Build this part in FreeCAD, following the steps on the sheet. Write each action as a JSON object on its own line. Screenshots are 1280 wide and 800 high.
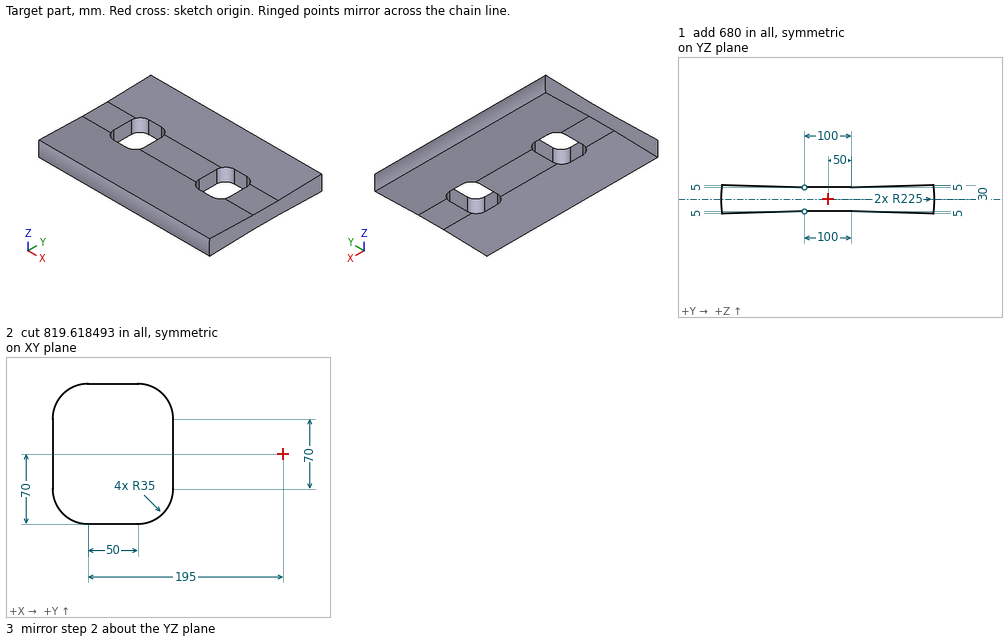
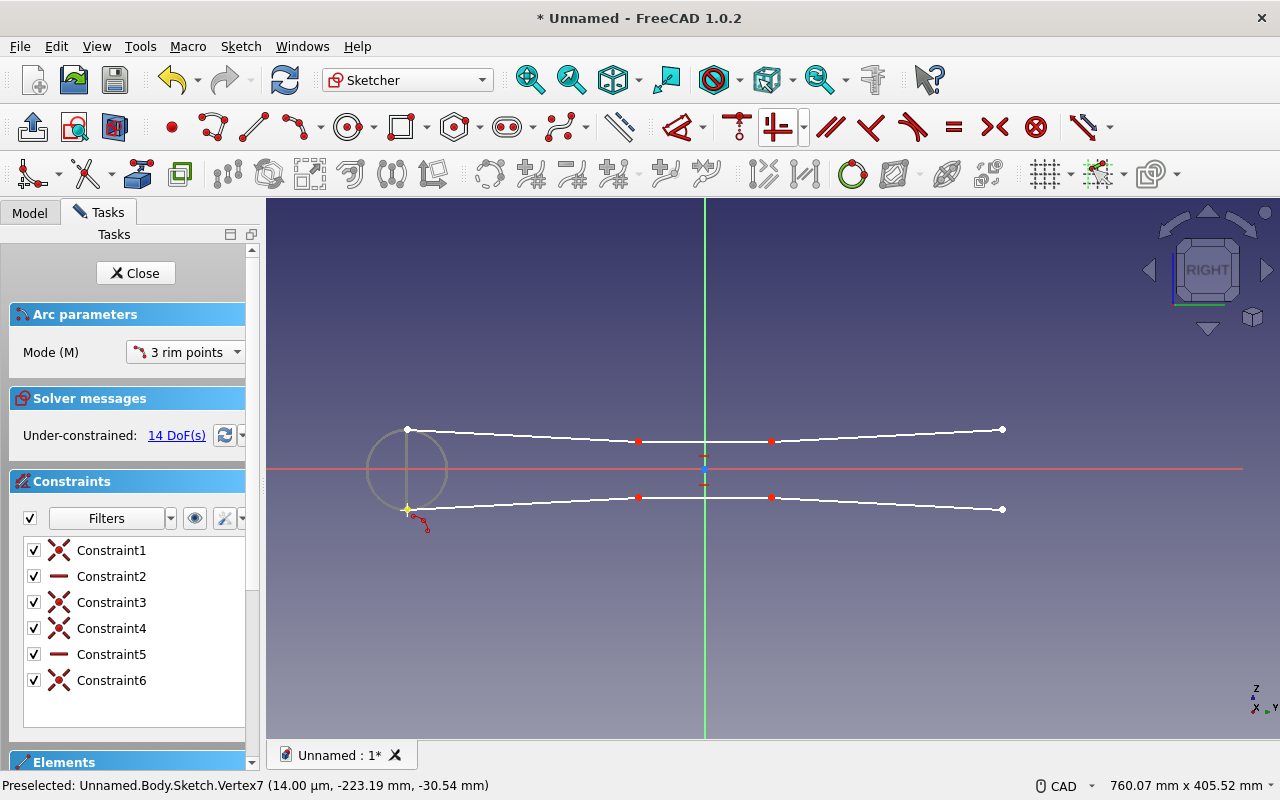
{"action": "scroll", "coordinate": [405, 461], "scroll_direction": "up", "scroll_amount": 10}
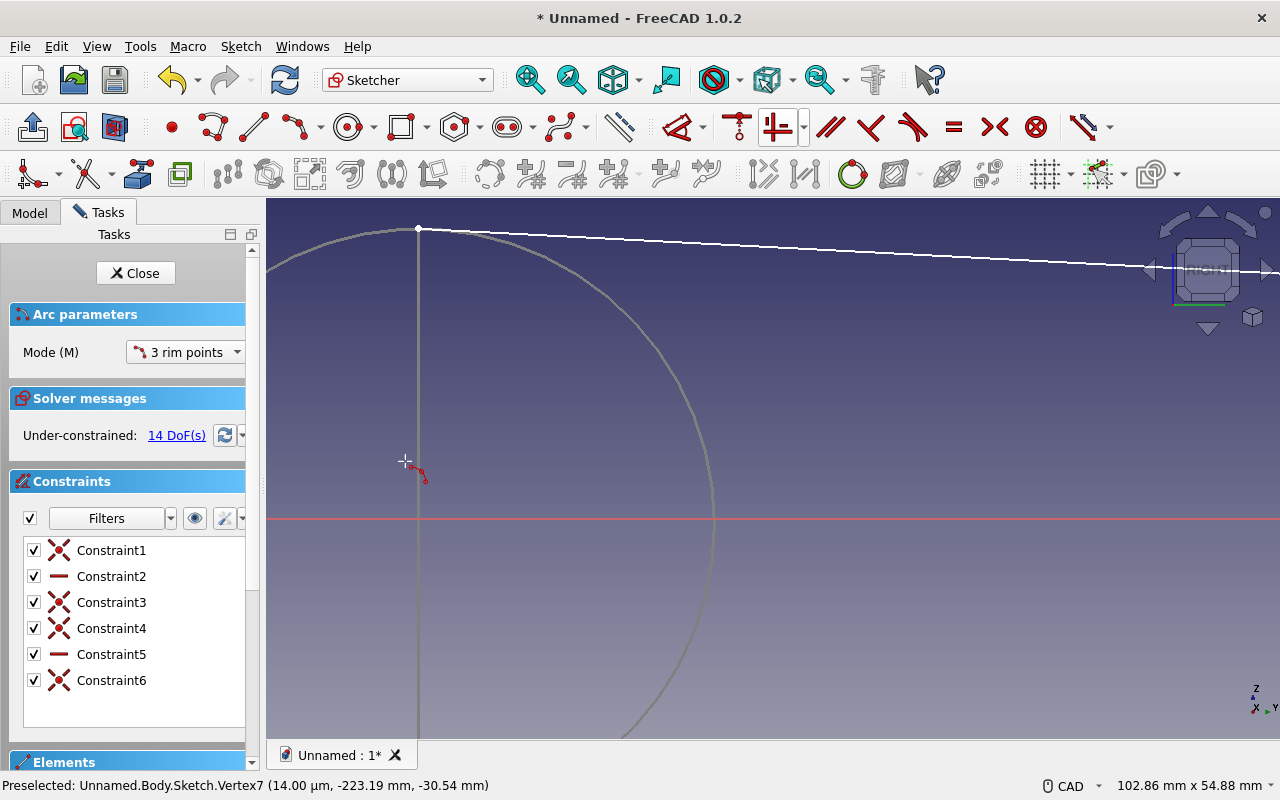
{"action": "left_click", "coordinate": [402, 460]}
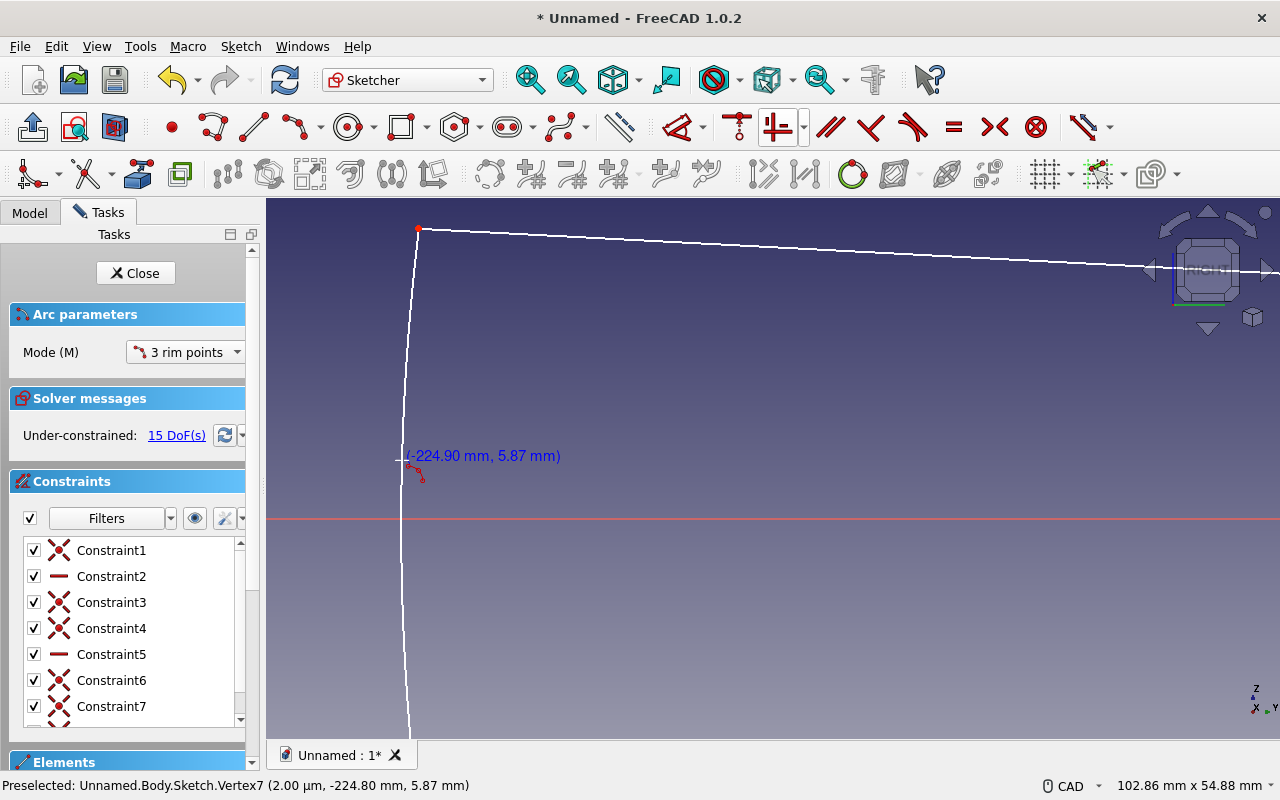
{"action": "scroll", "coordinate": [405, 461], "scroll_direction": "down", "scroll_amount": 10}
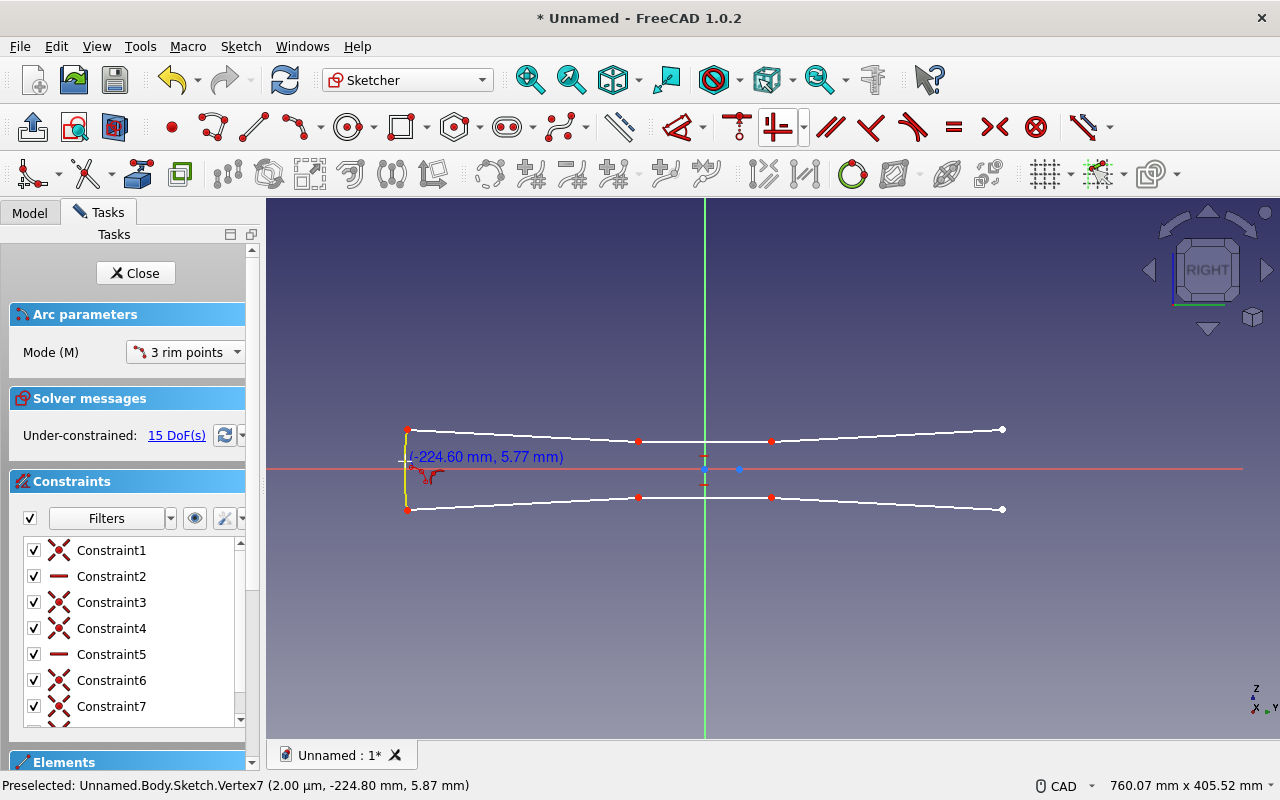
{"action": "left_click", "coordinate": [1002, 510]}
{"action": "left_click", "coordinate": [1002, 430]}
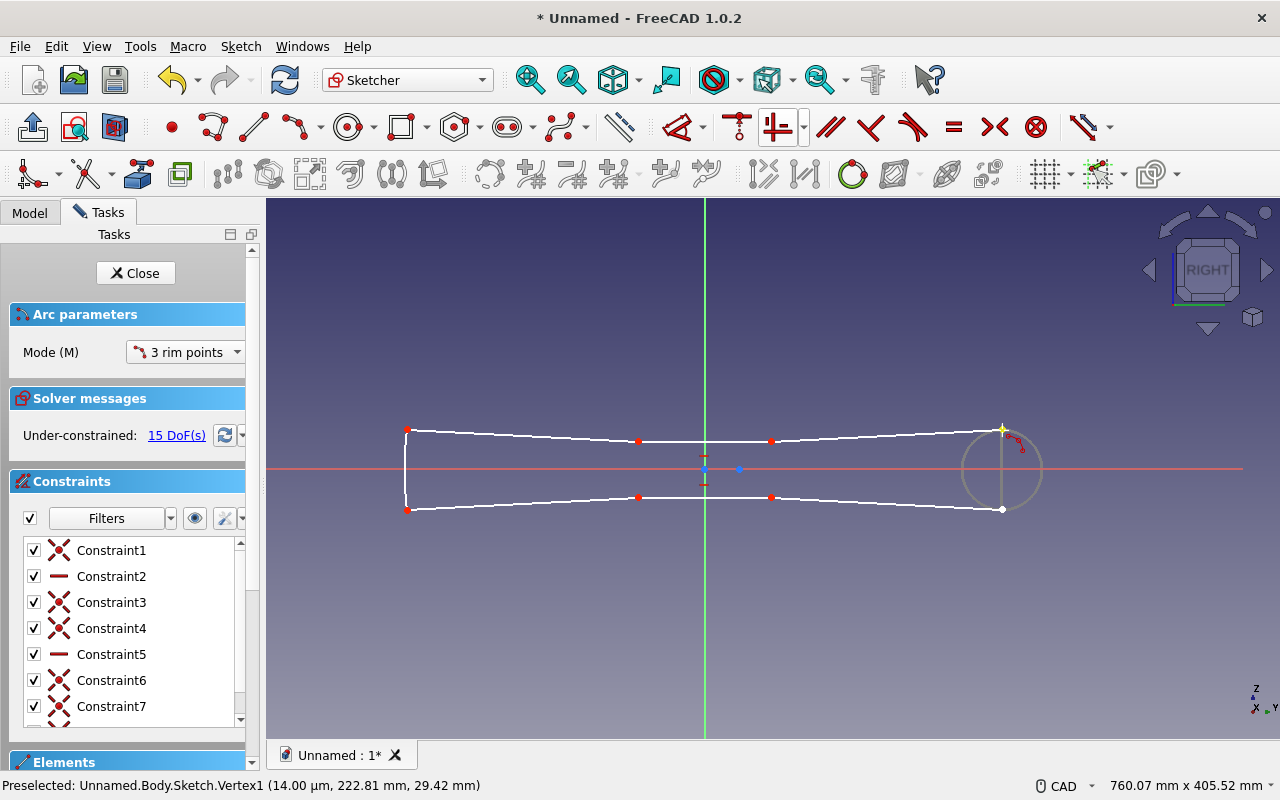
{"action": "scroll", "coordinate": [1005, 477], "scroll_direction": "up", "scroll_amount": 10}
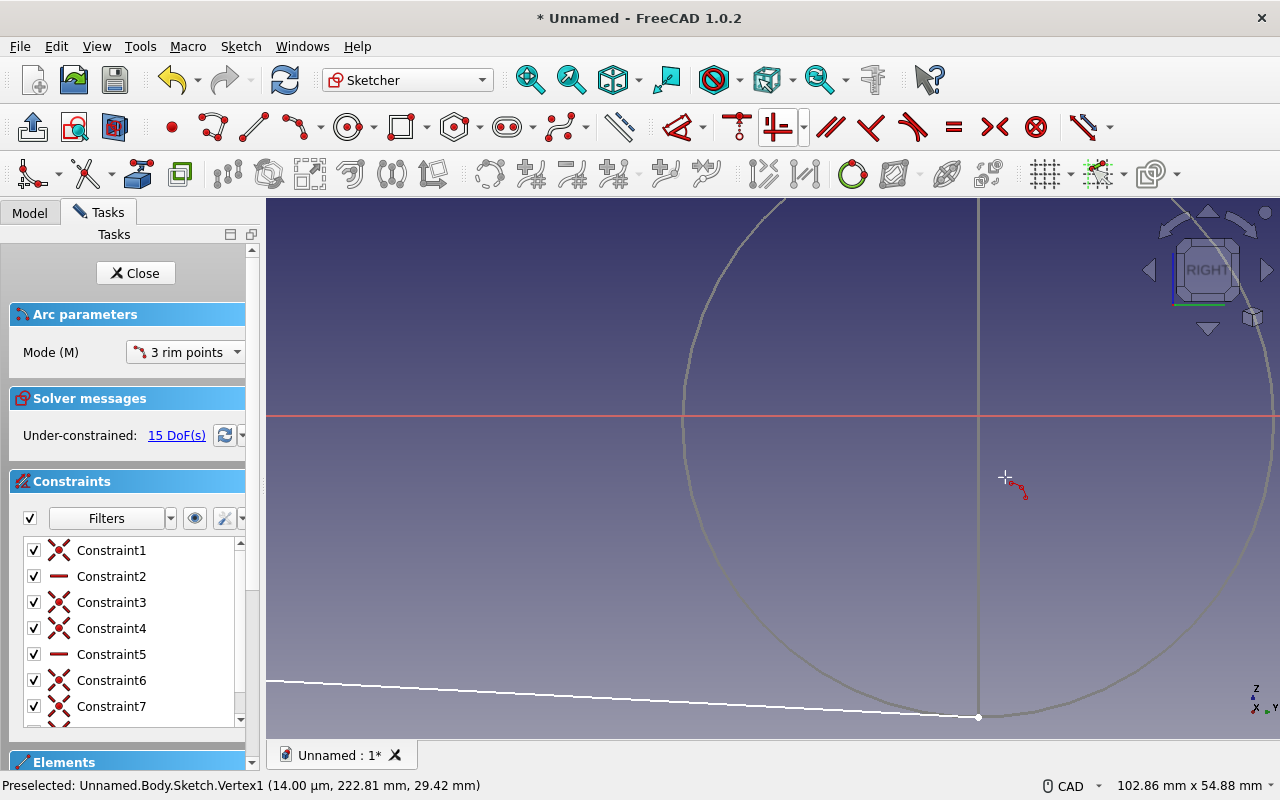
{"action": "left_click", "coordinate": [999, 476]}
{"action": "key", "text": "Escape"}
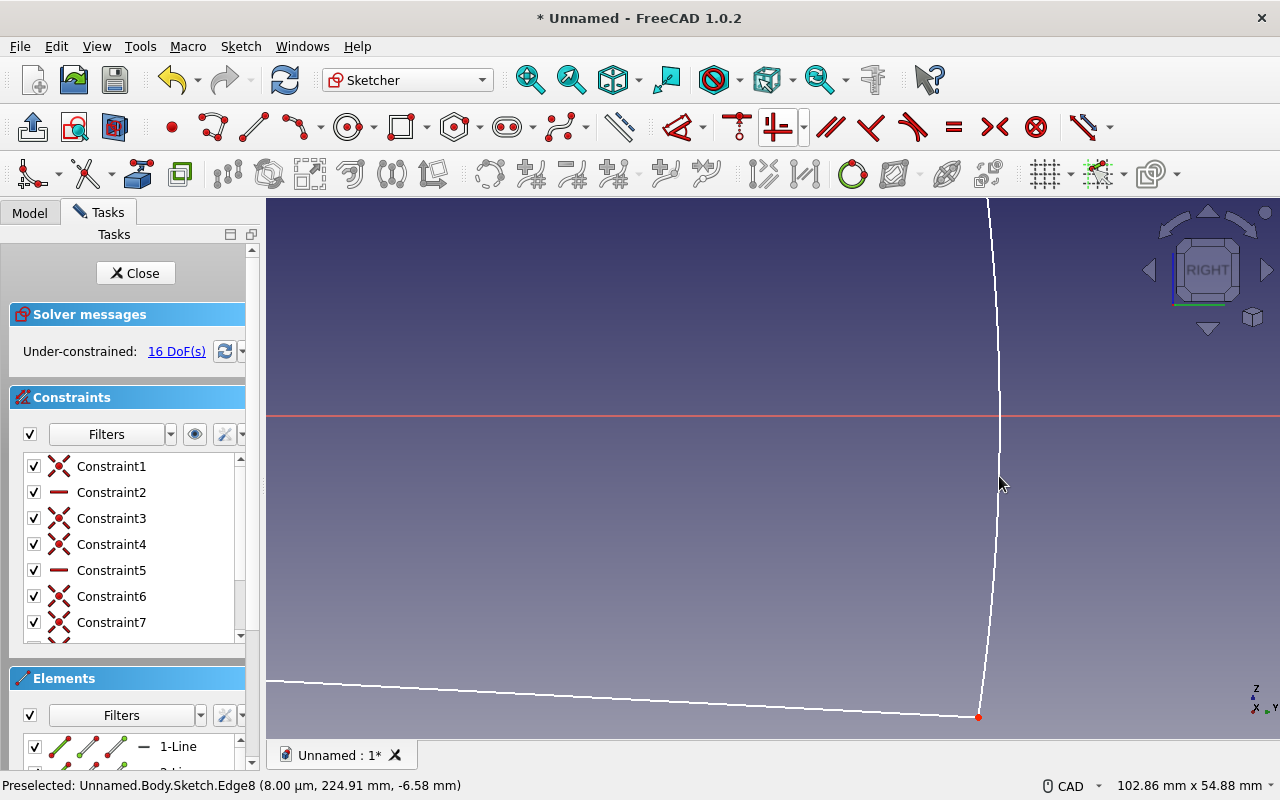
{"action": "scroll", "coordinate": [1005, 477], "scroll_direction": "down", "scroll_amount": 10}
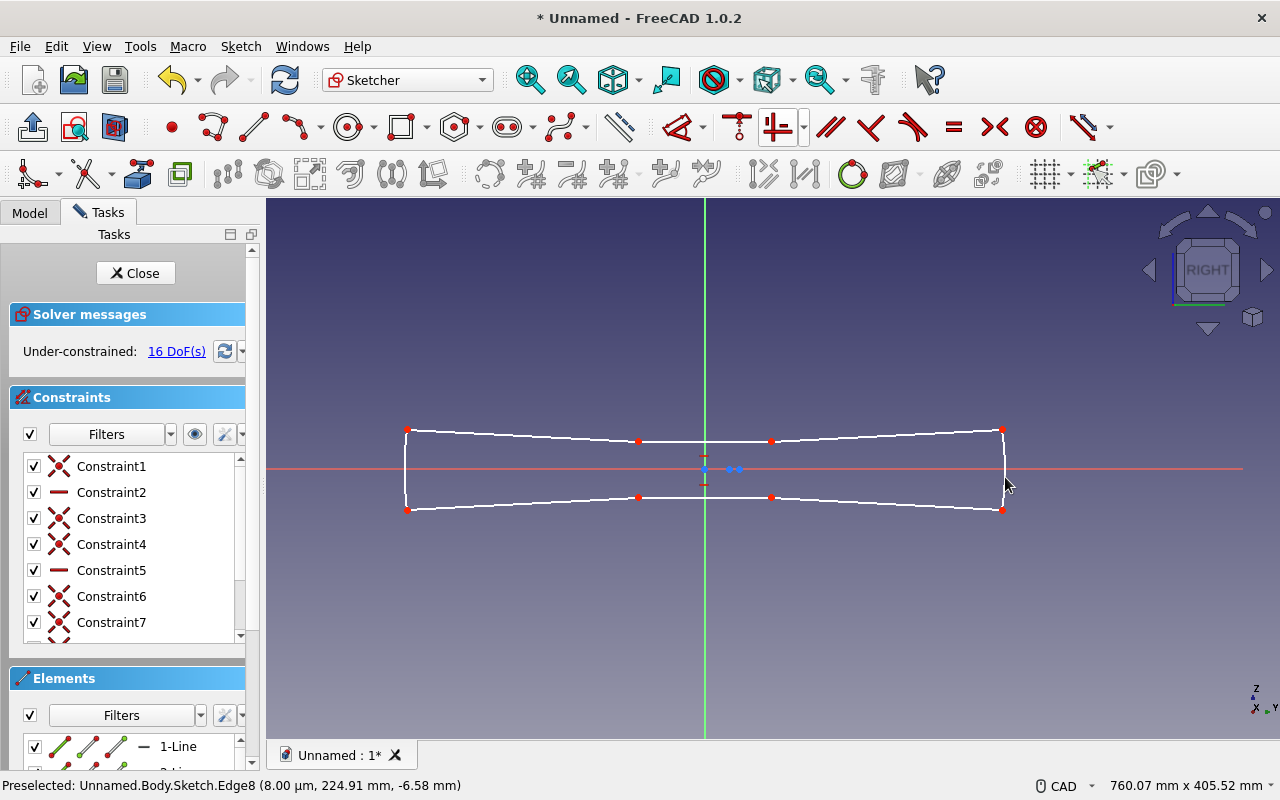
{"action": "left_click", "coordinate": [405, 454]}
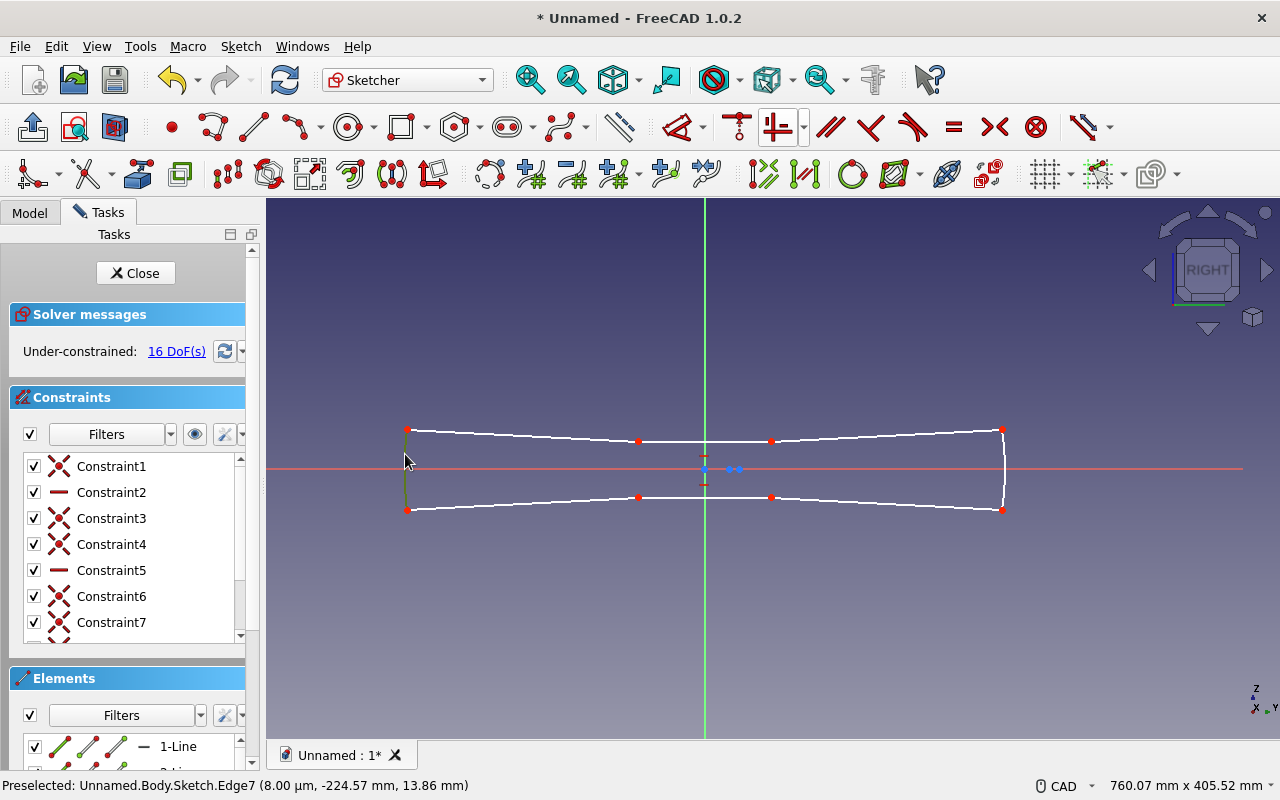
{"action": "left_click", "coordinate": [1004, 486]}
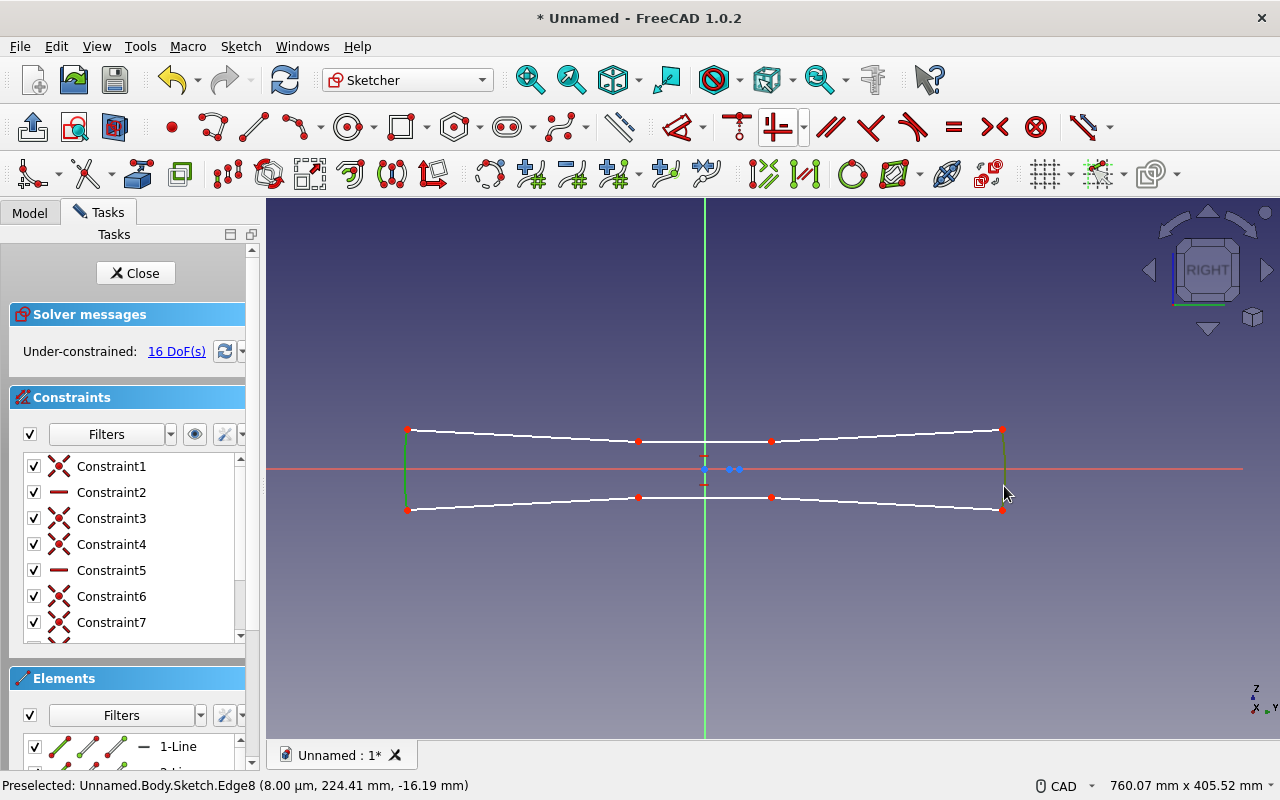
{"action": "key", "text": "c"}